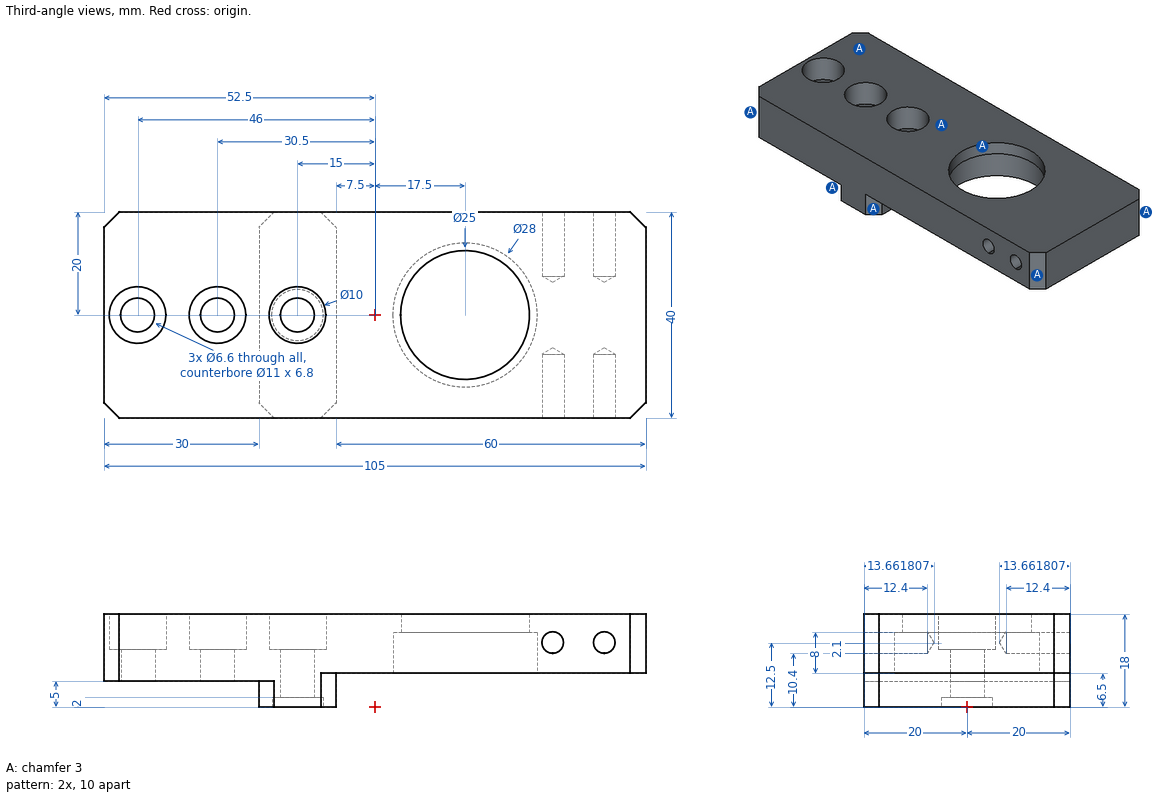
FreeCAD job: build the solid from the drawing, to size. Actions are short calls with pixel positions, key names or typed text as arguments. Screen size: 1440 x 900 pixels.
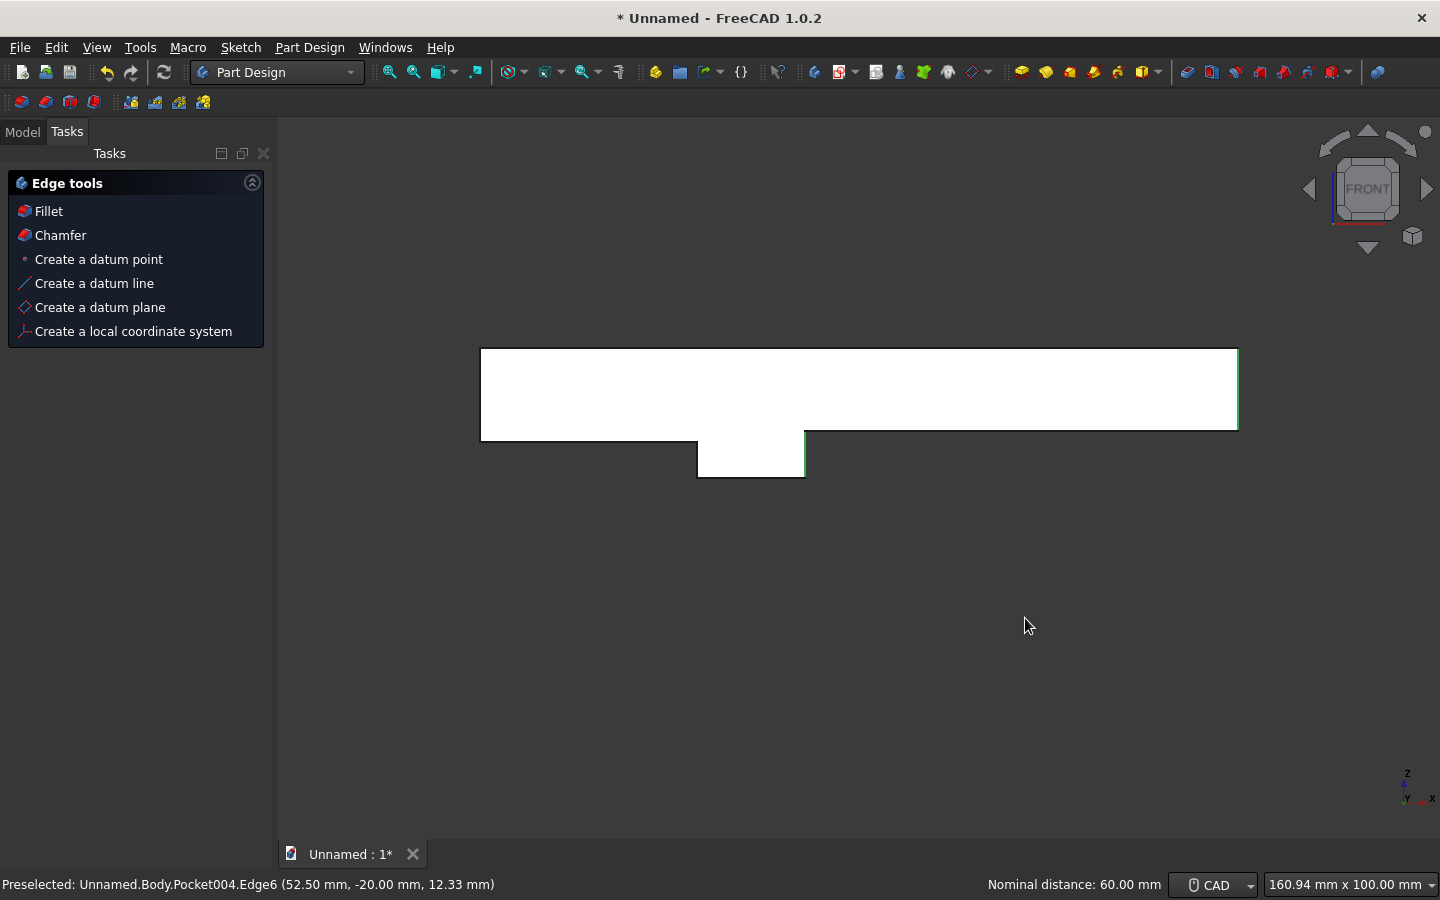
click(697, 459, ctrl)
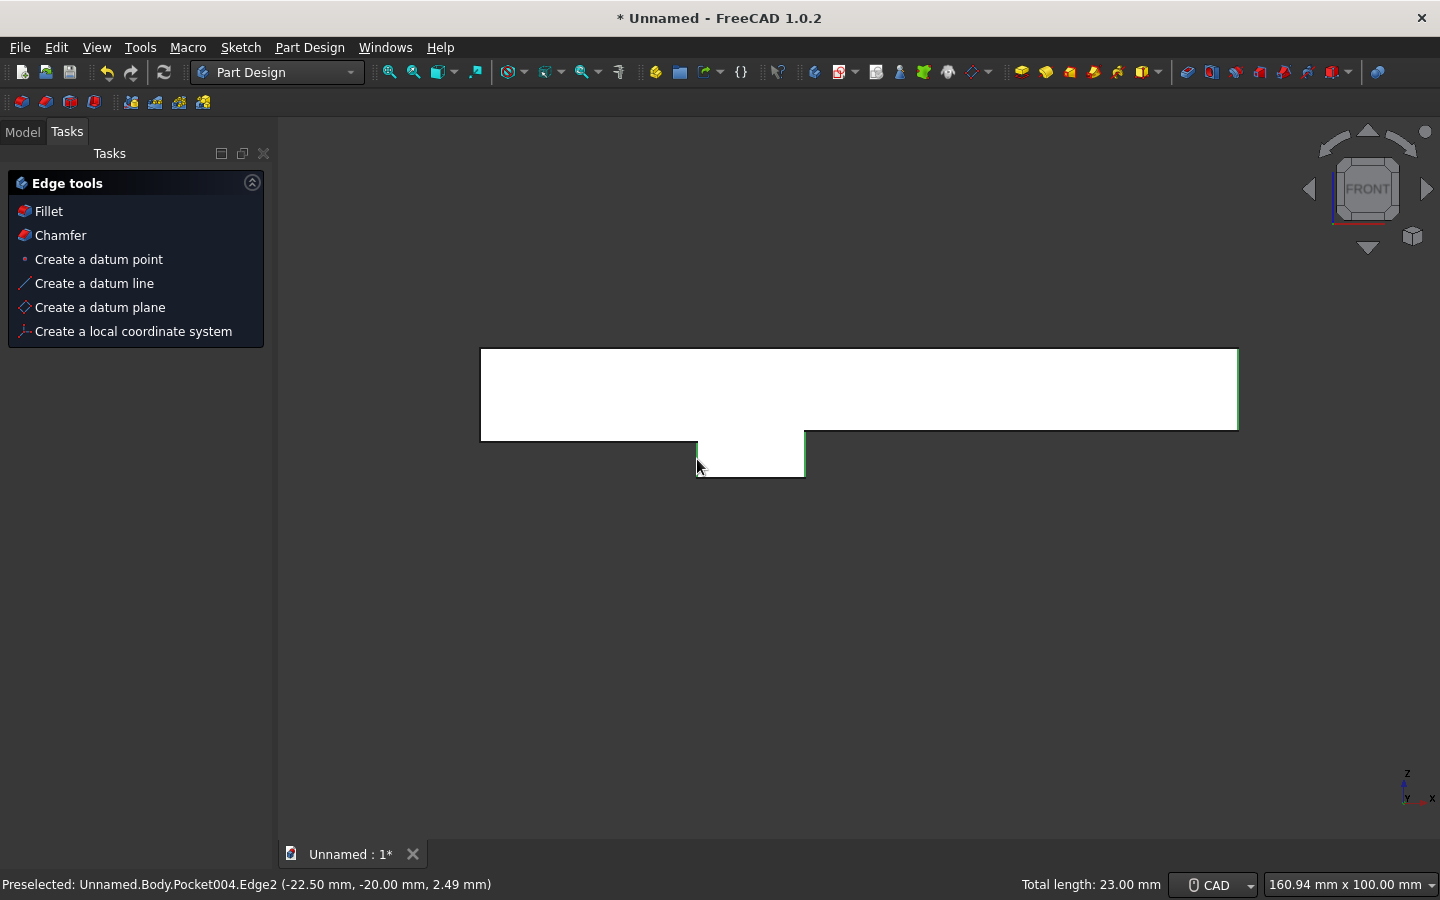
click(480, 394, ctrl)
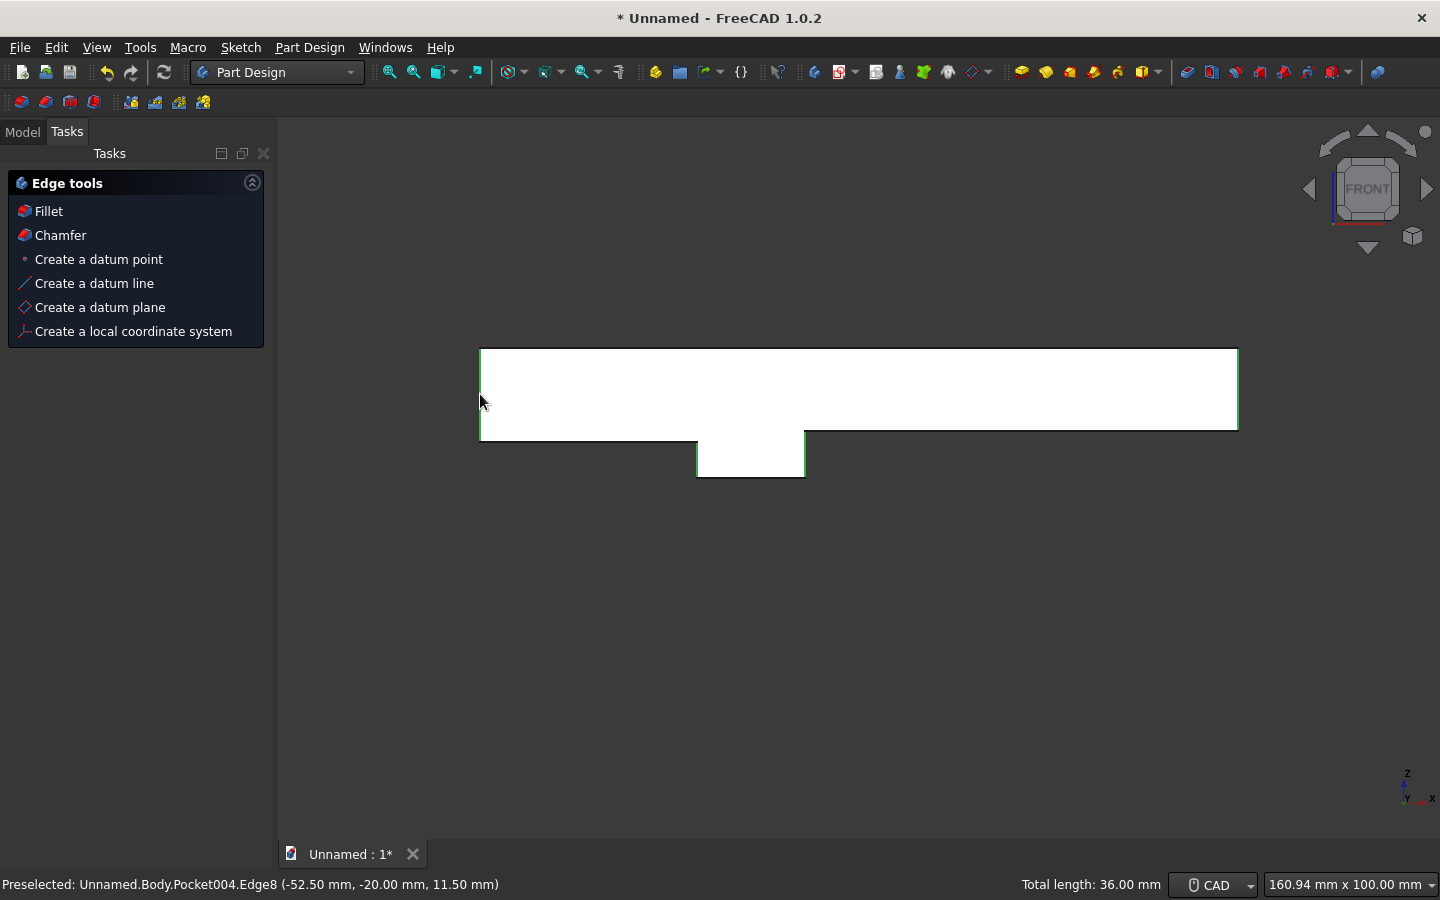
key(3)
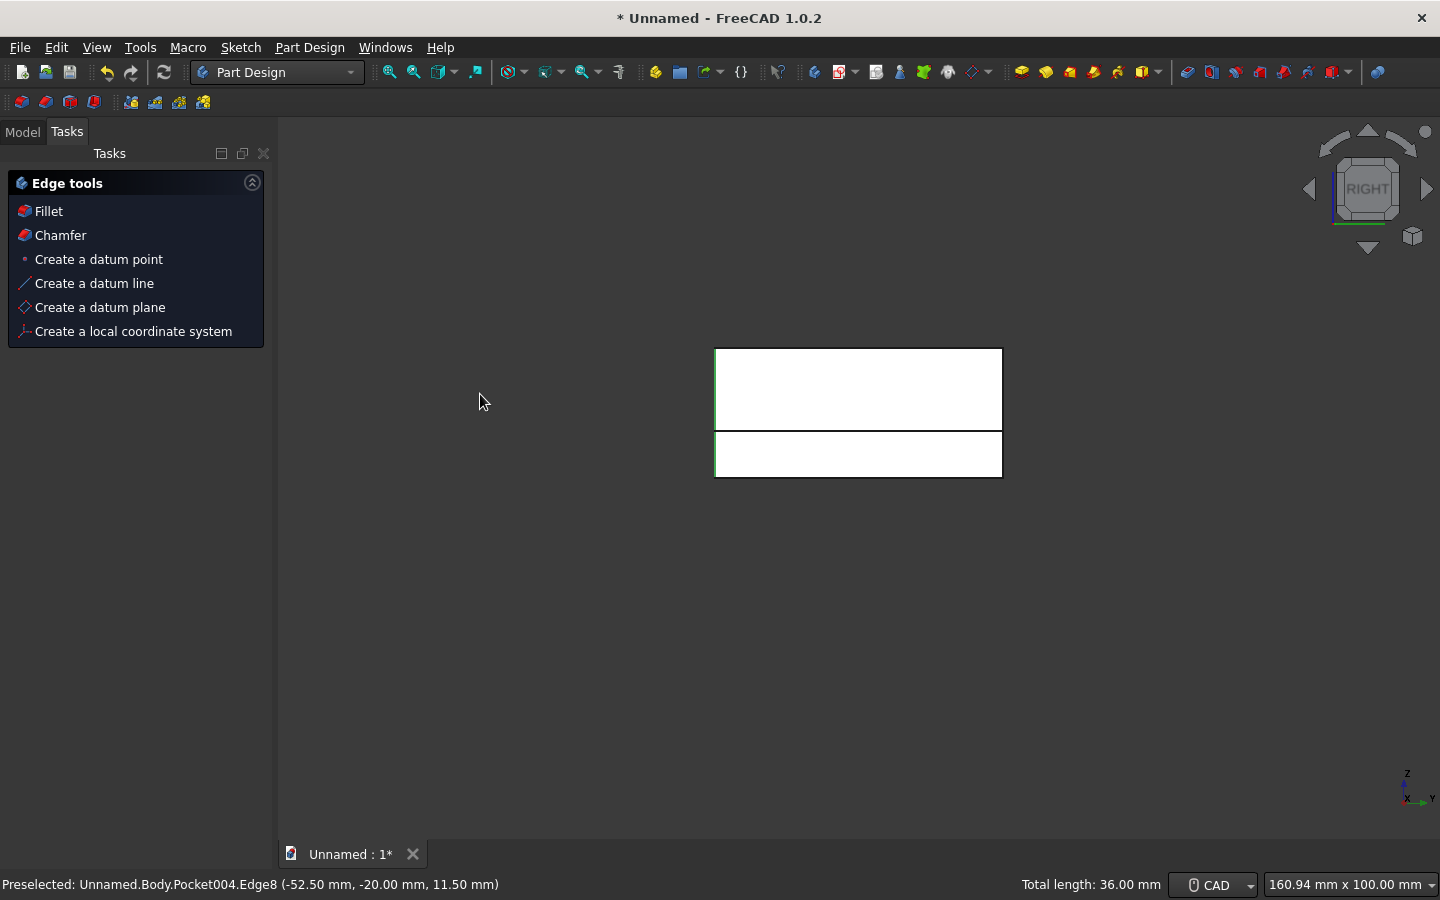
click(390, 72)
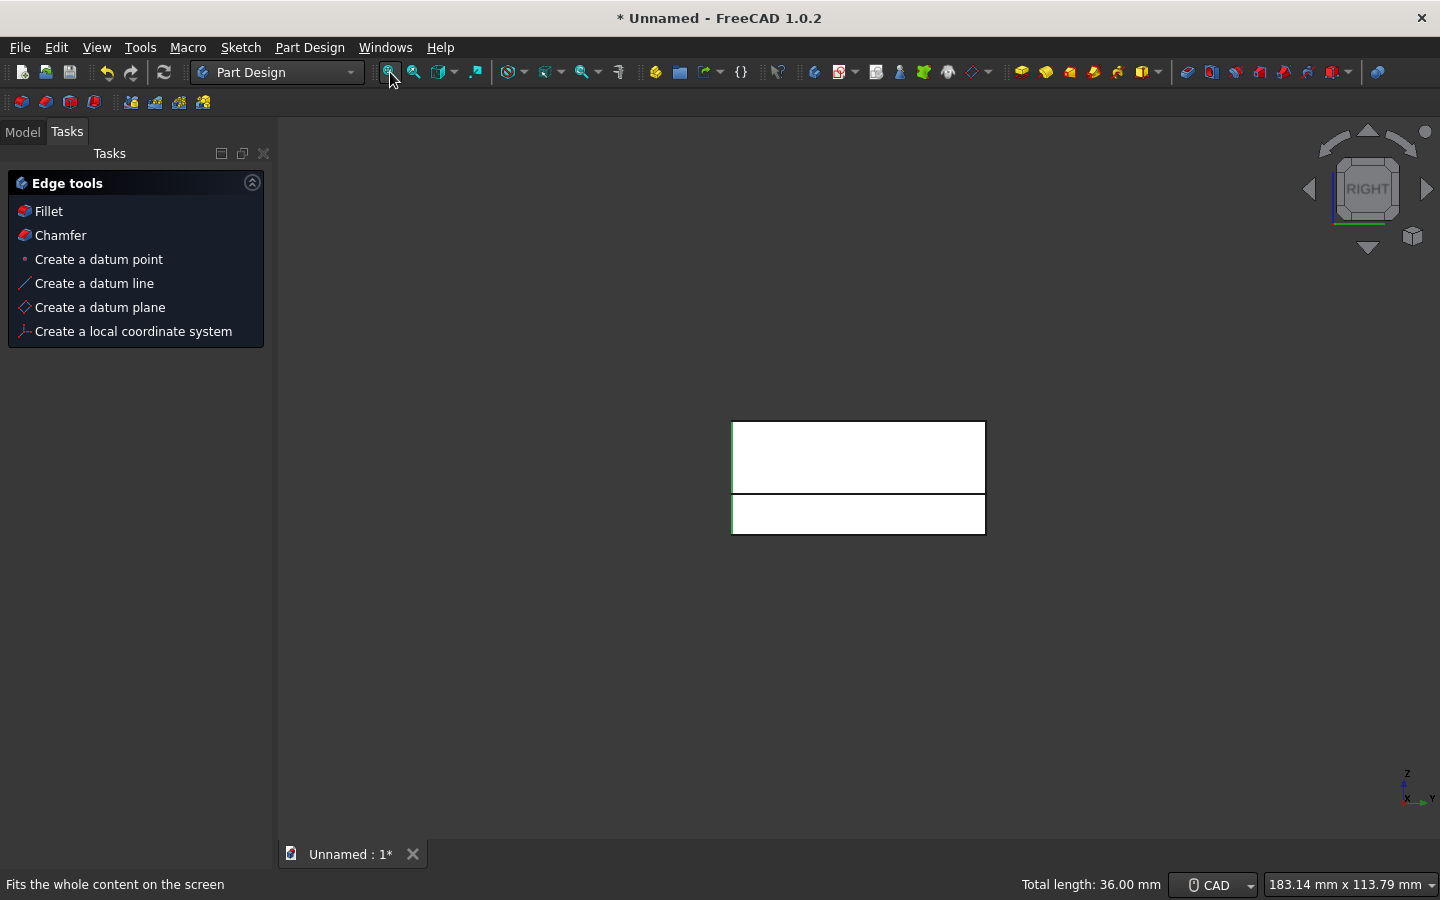
click(986, 513, ctrl)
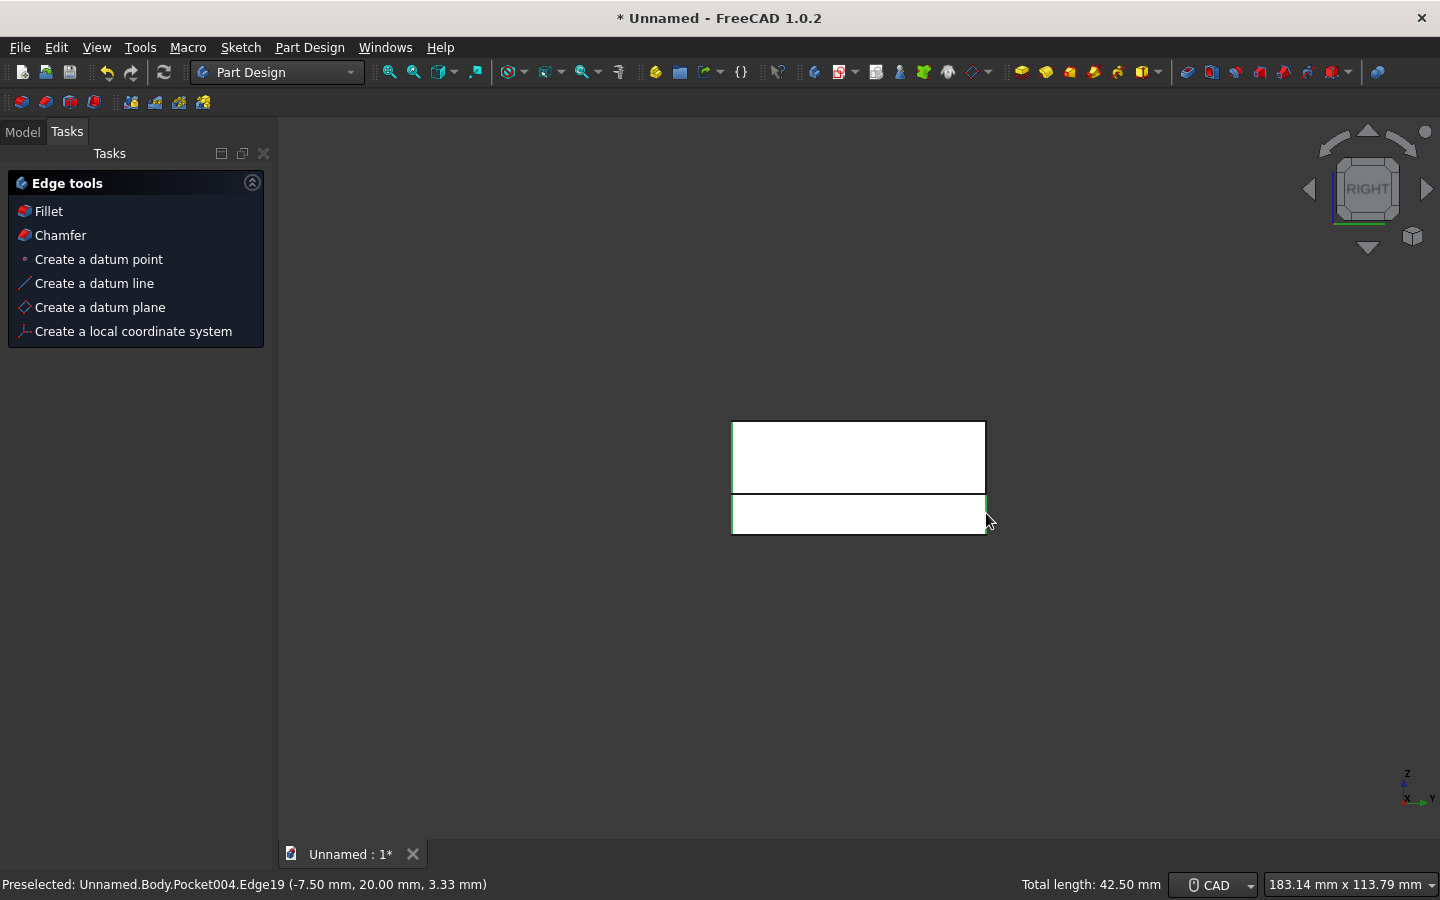
click(986, 456, ctrl)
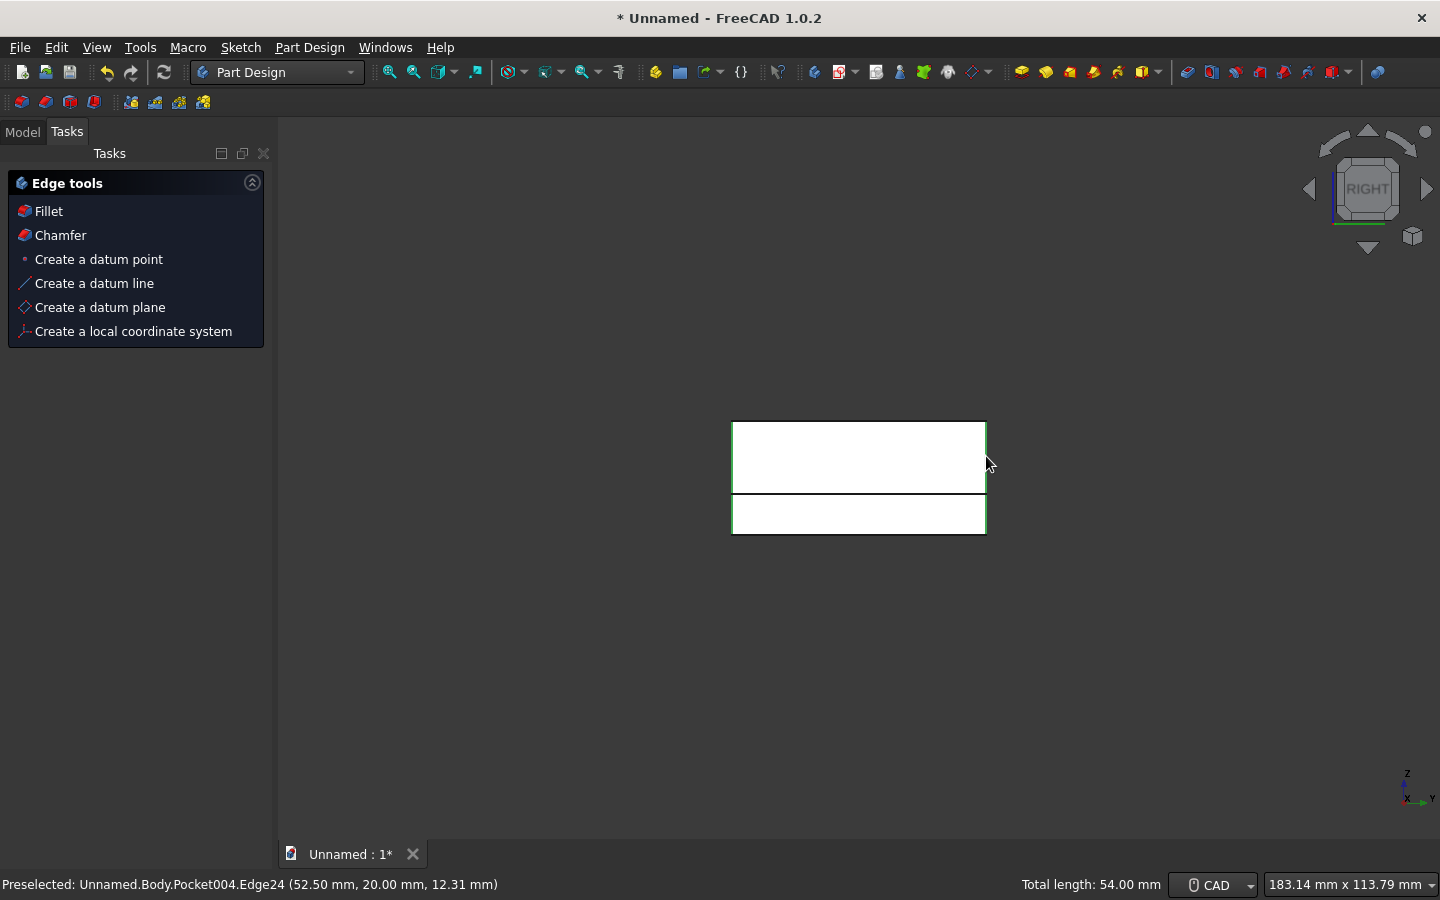
key(5)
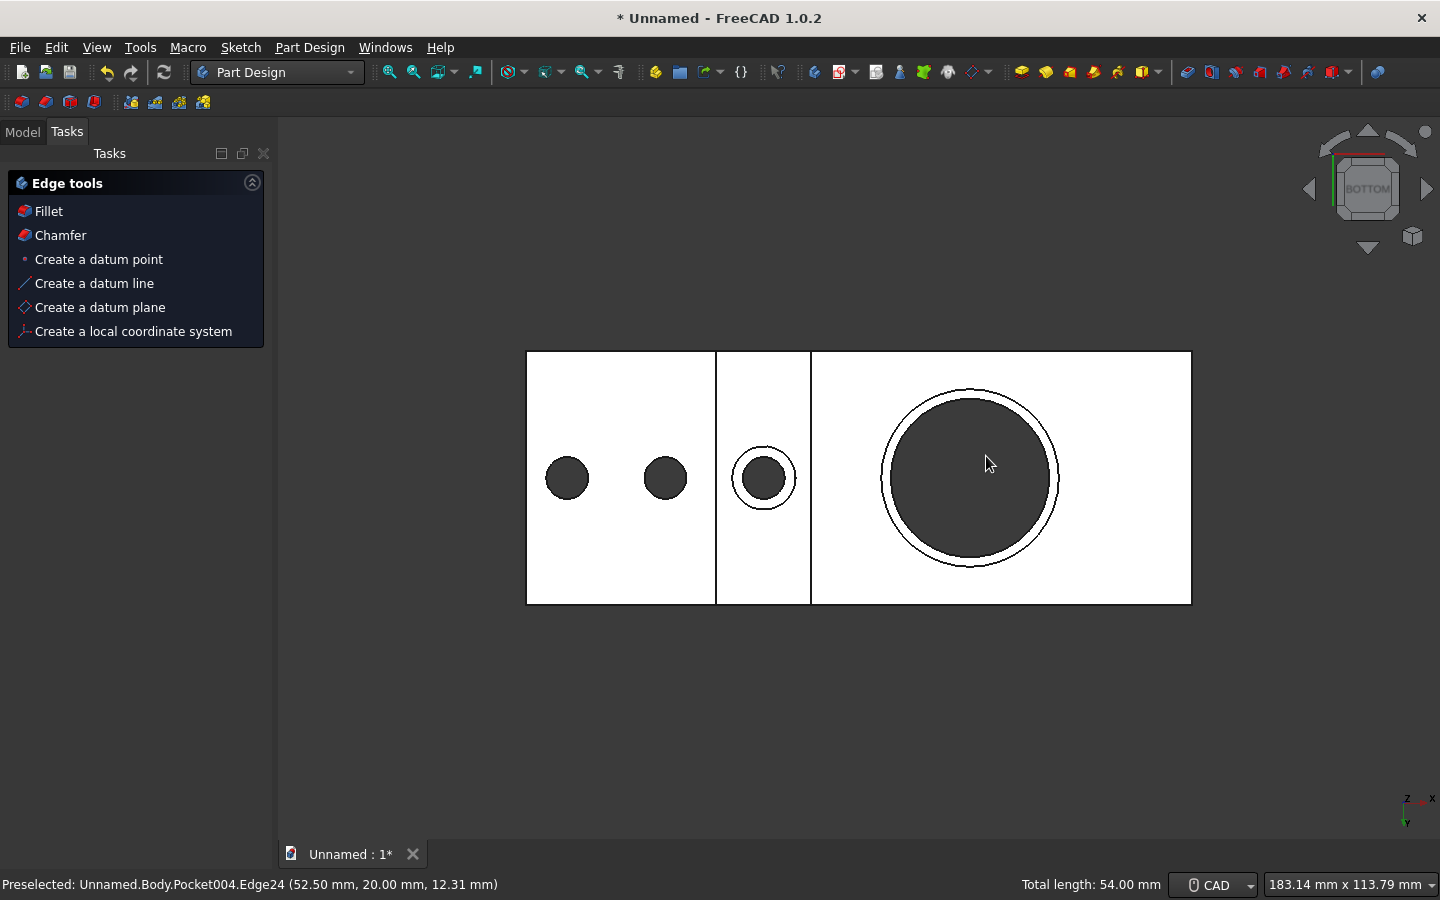
key(4)